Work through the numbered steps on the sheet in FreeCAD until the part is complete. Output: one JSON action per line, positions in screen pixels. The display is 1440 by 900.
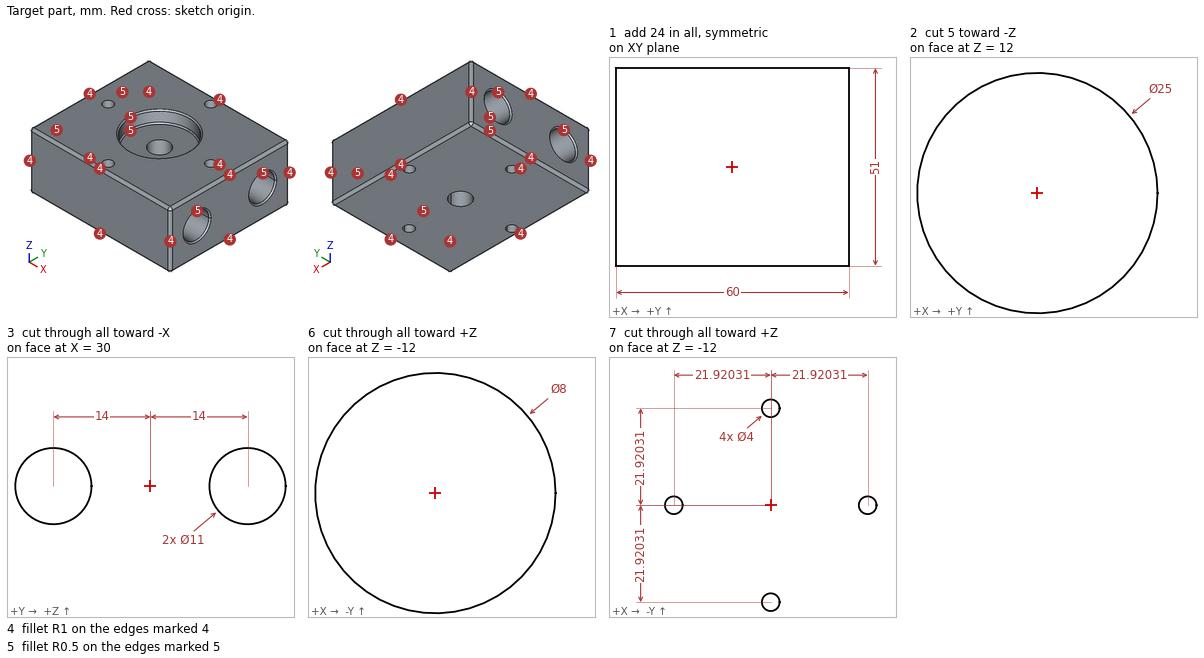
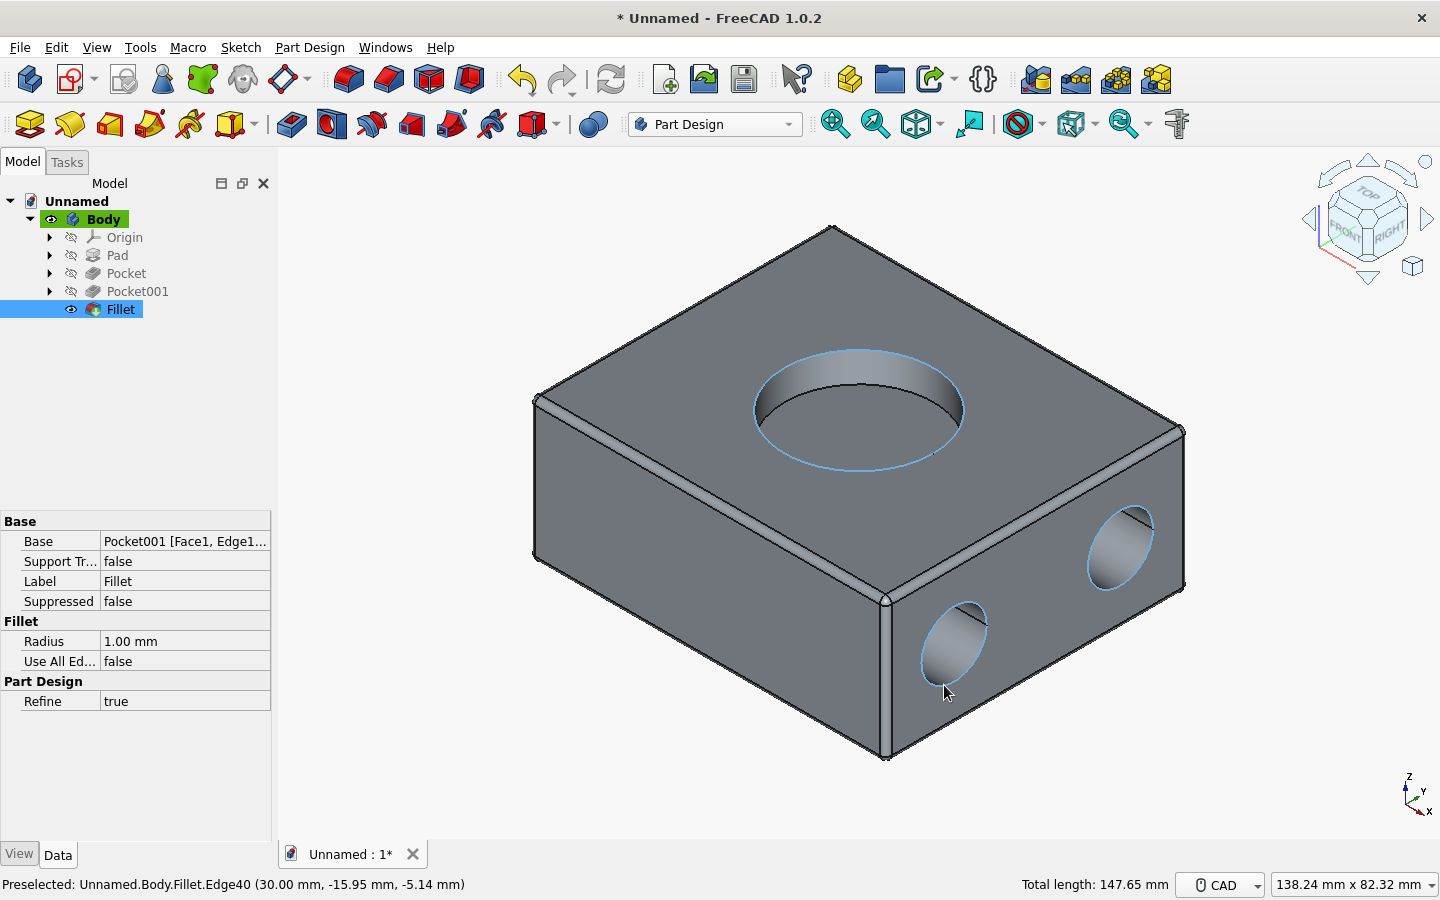
{"action": "key", "text": "2"}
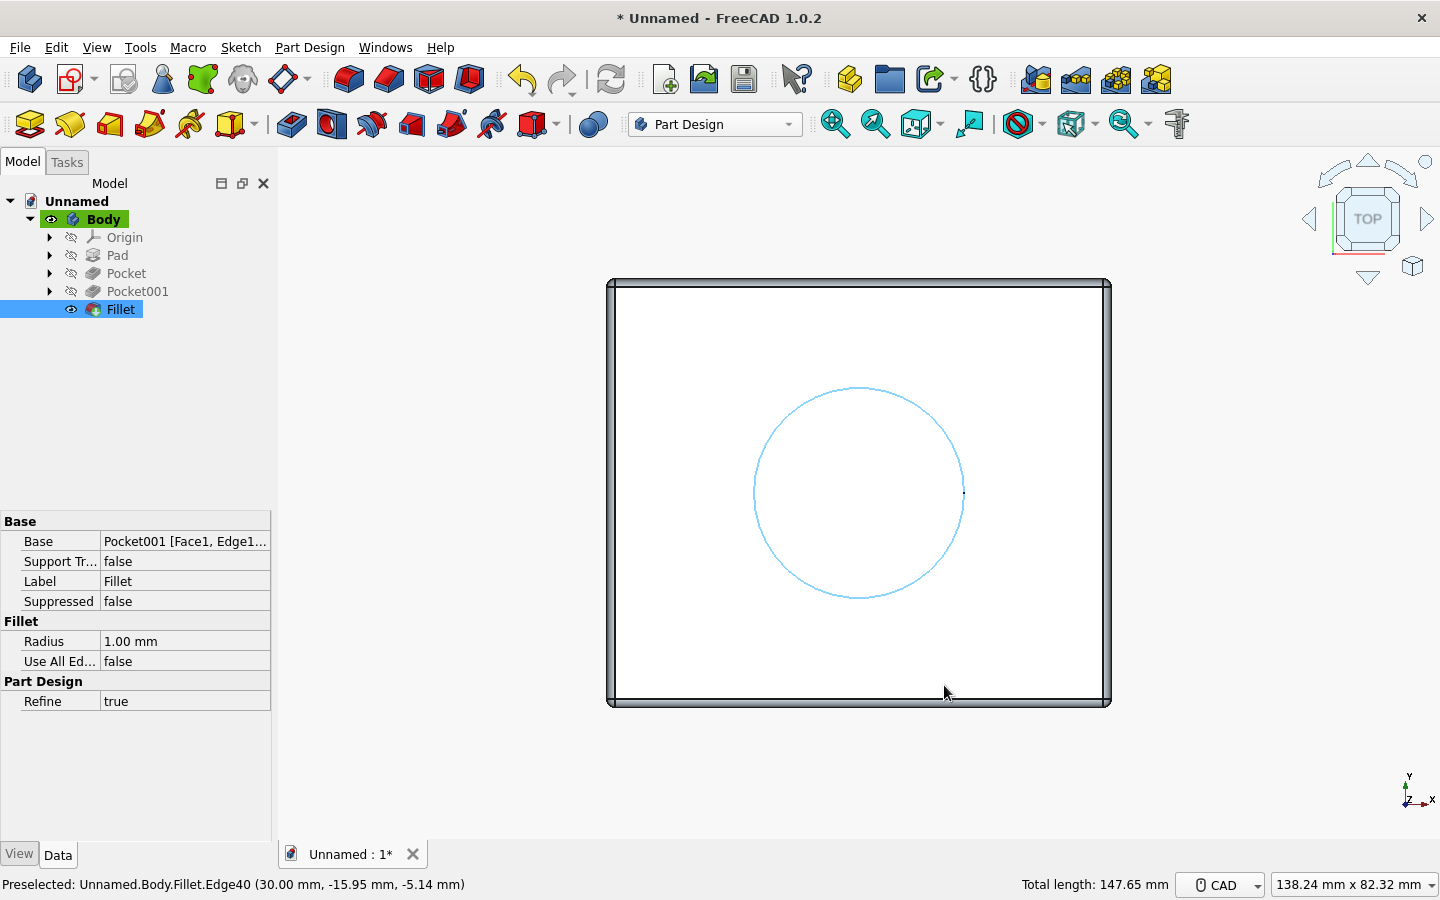
{"action": "key", "text": "1"}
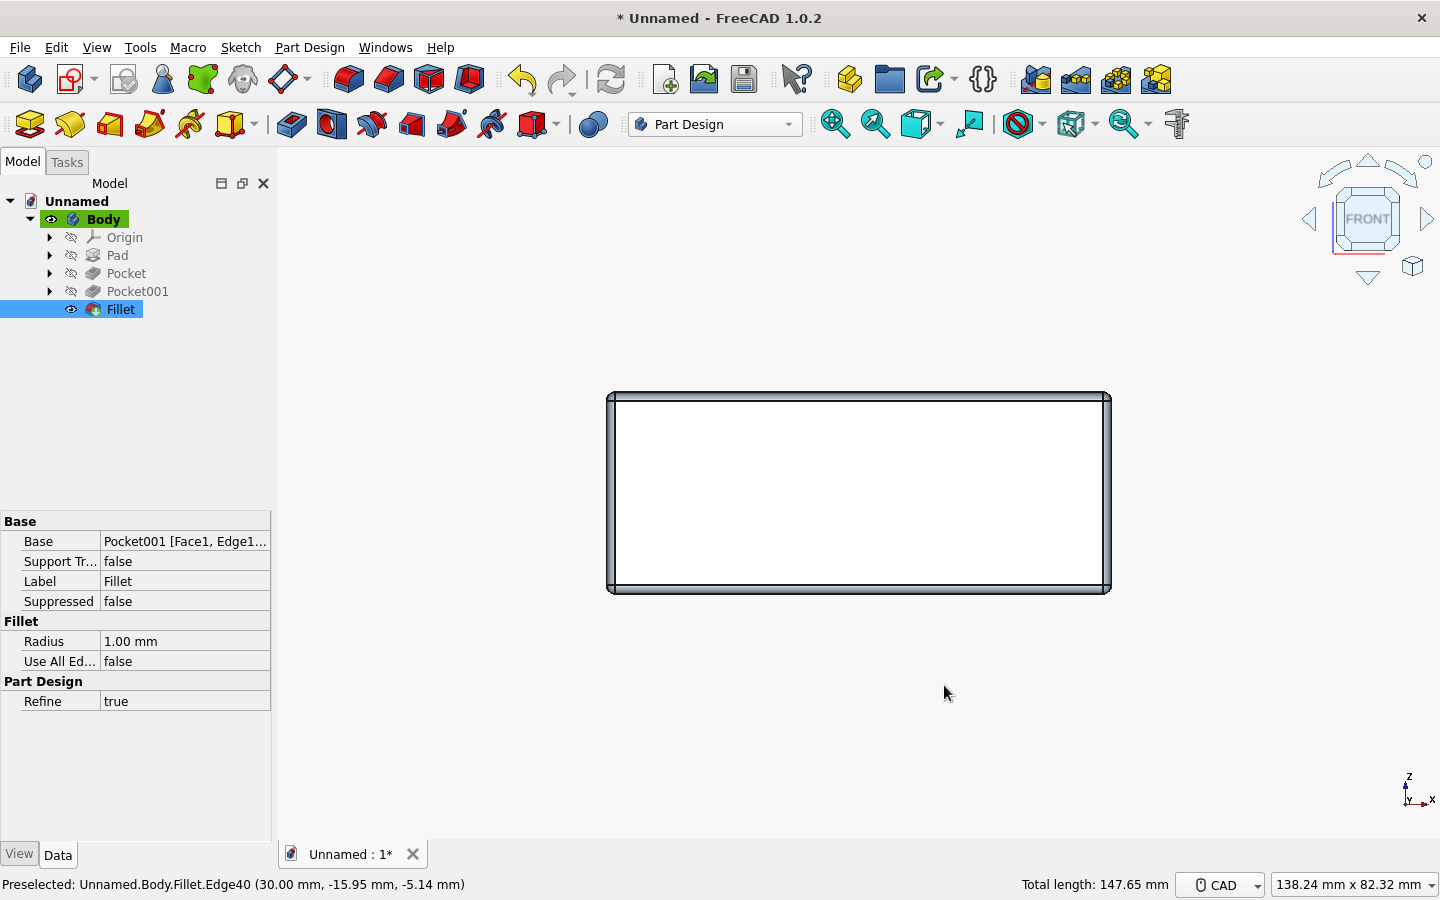
{"action": "left_click", "coordinate": [836, 124]}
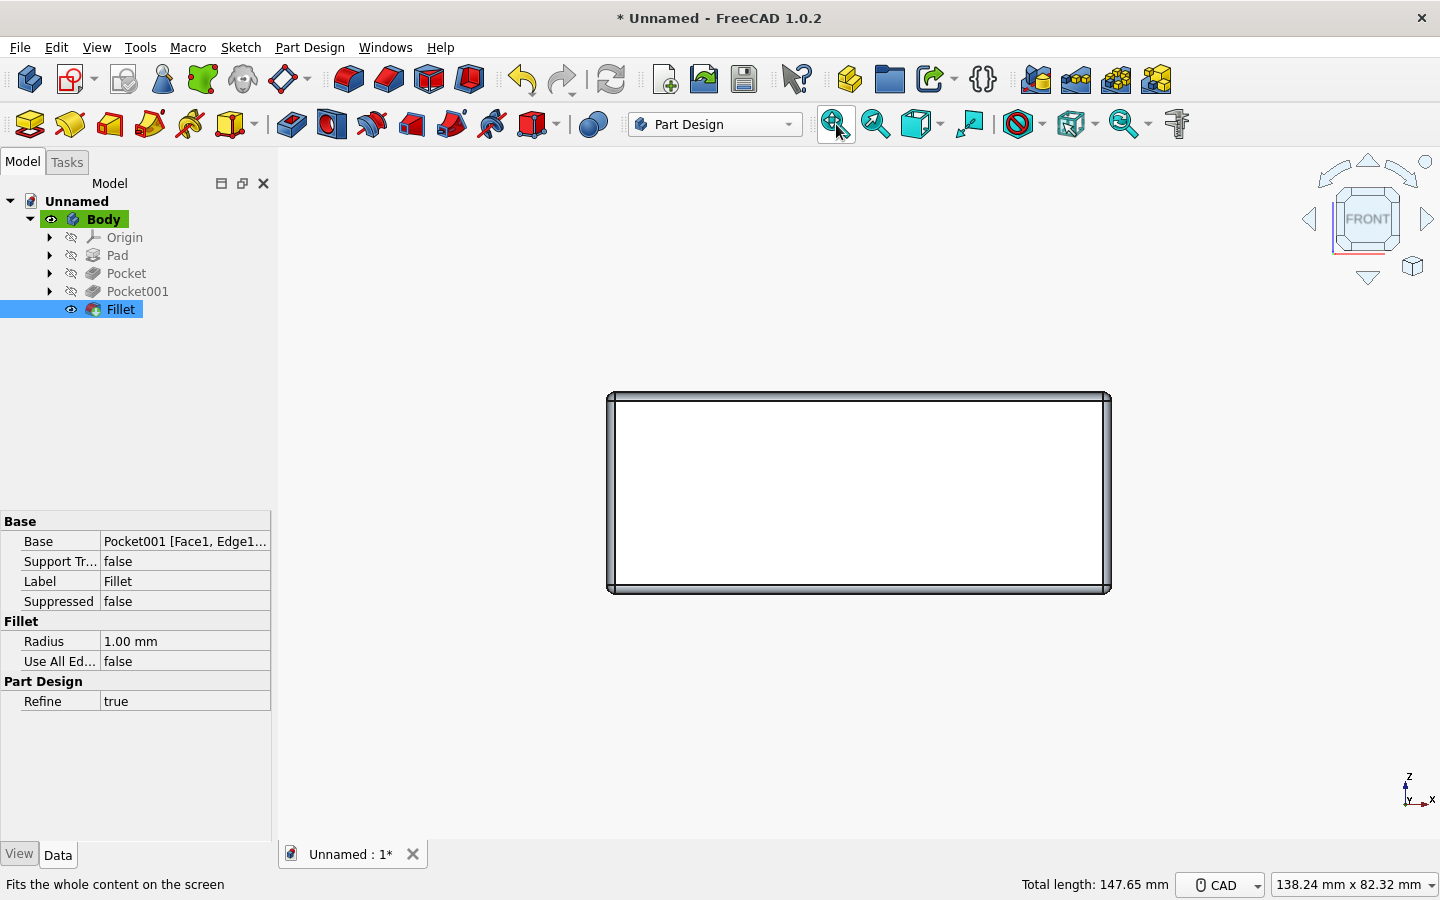
{"action": "key", "text": "3"}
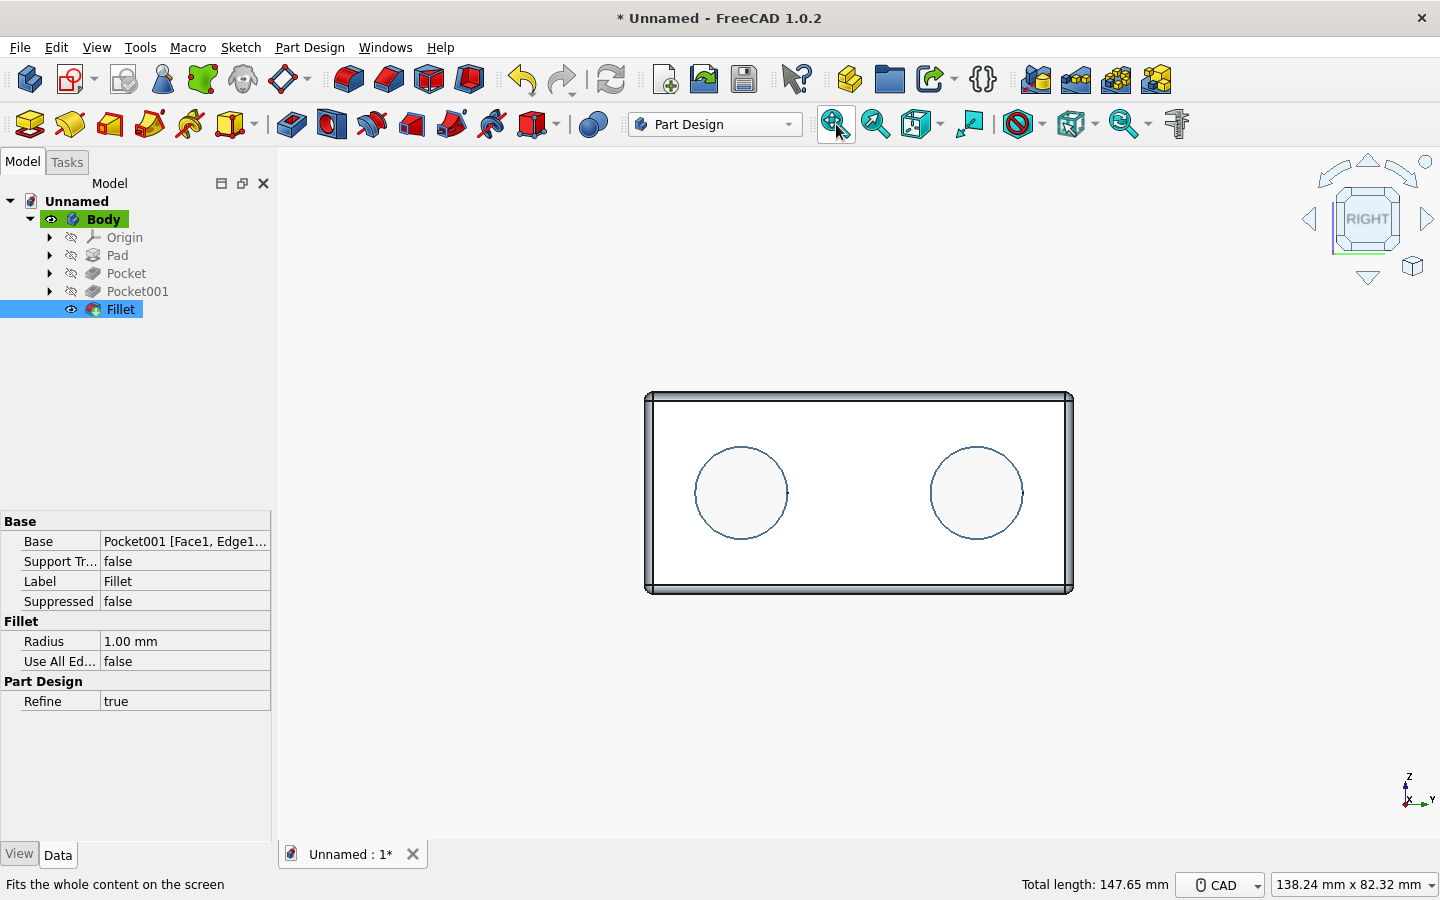
{"action": "left_click", "coordinate": [836, 124]}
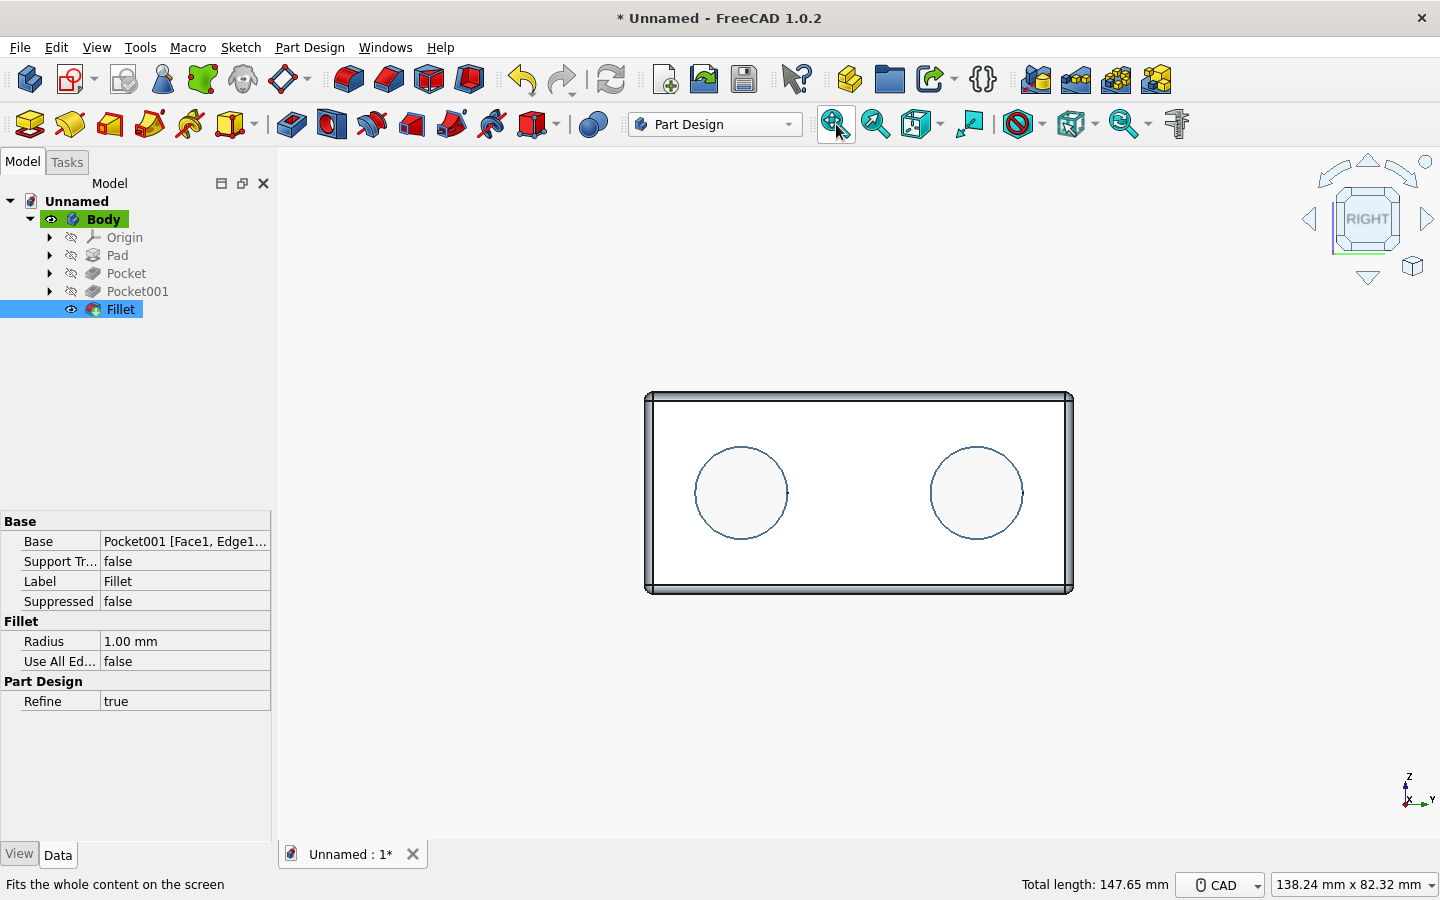
{"action": "key", "text": "5"}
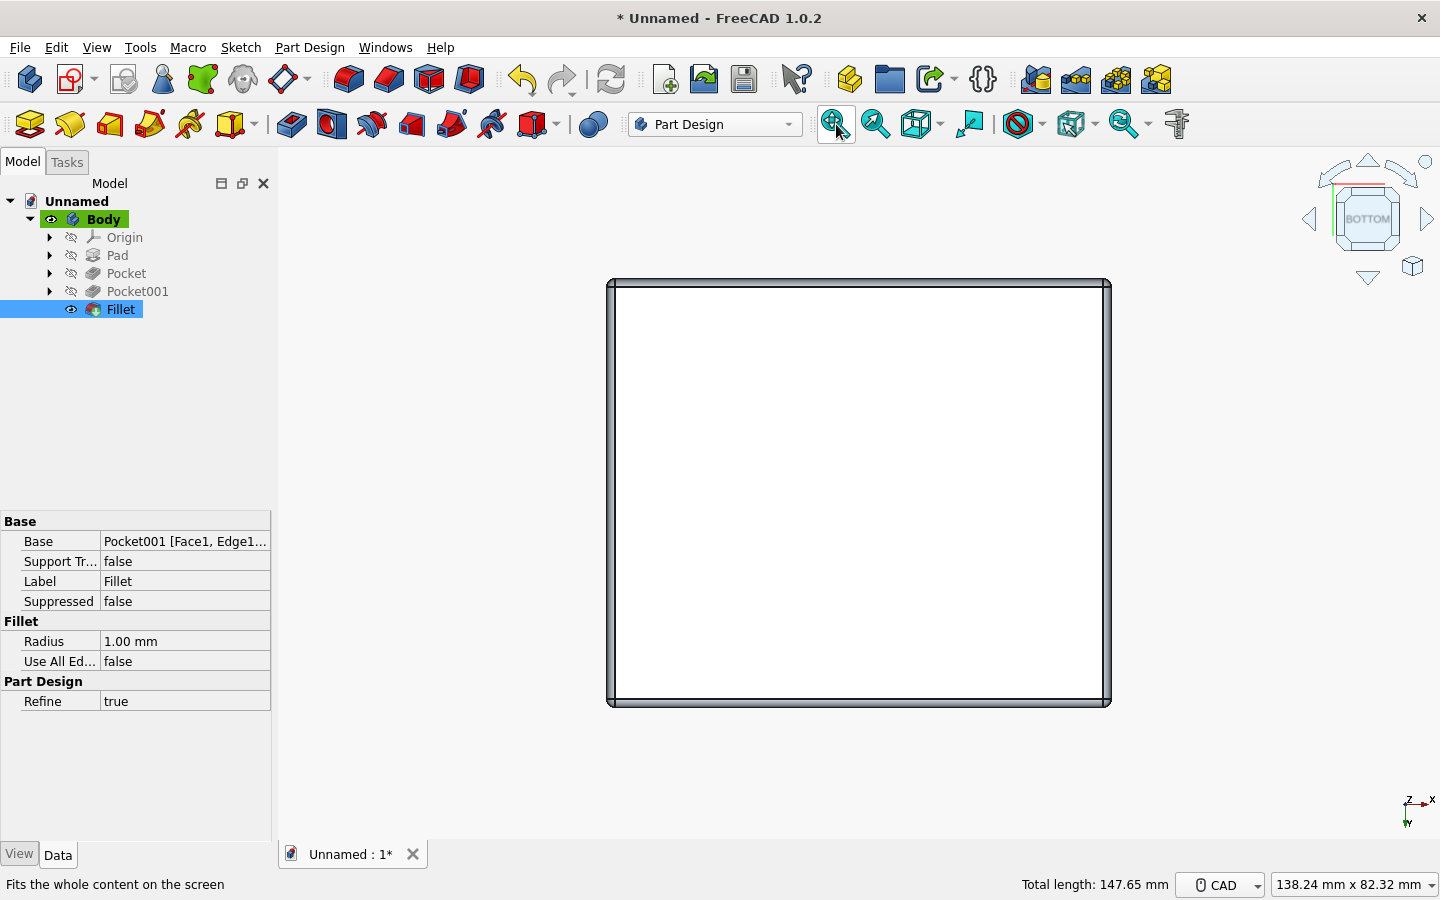
{"action": "key", "text": "4"}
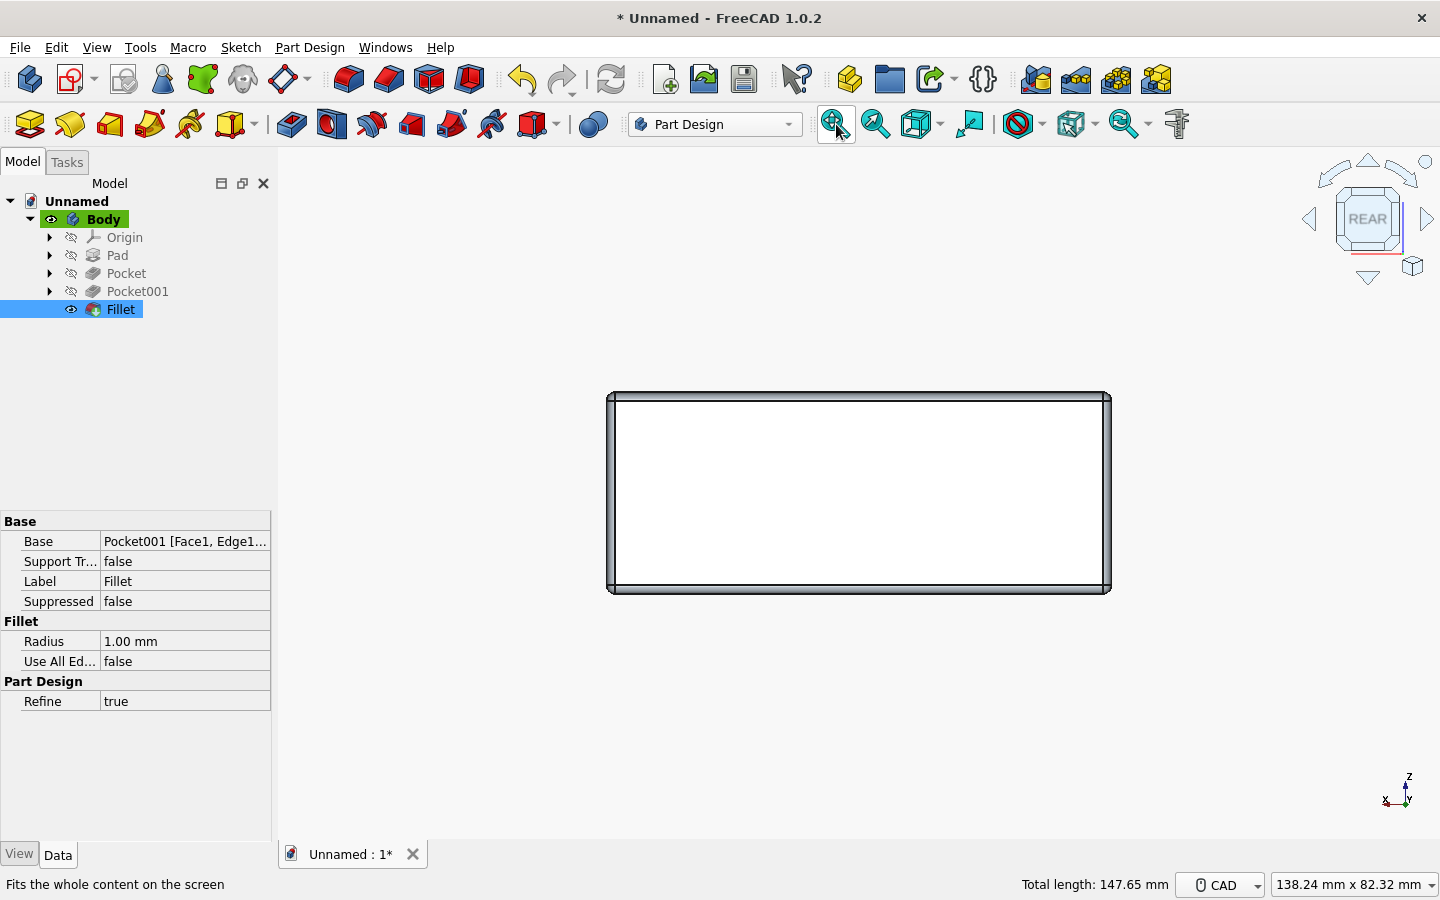
{"action": "left_click", "coordinate": [836, 124]}